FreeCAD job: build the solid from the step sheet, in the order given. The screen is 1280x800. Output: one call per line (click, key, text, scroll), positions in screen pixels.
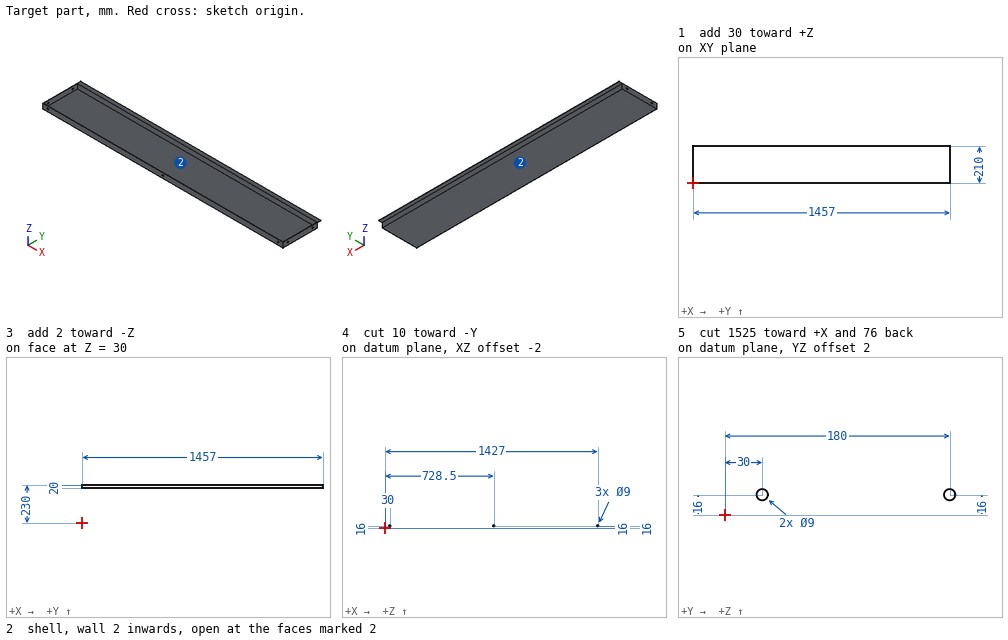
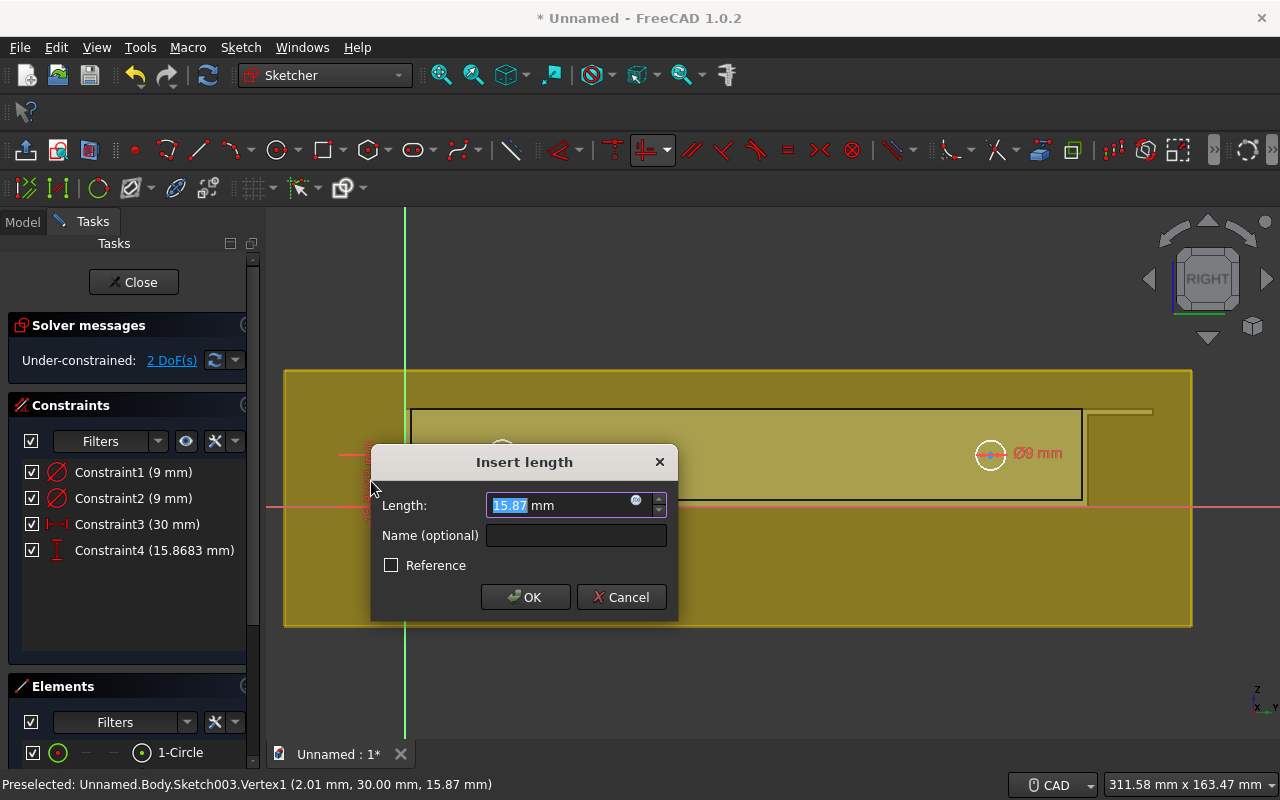
text(16)
key(Return)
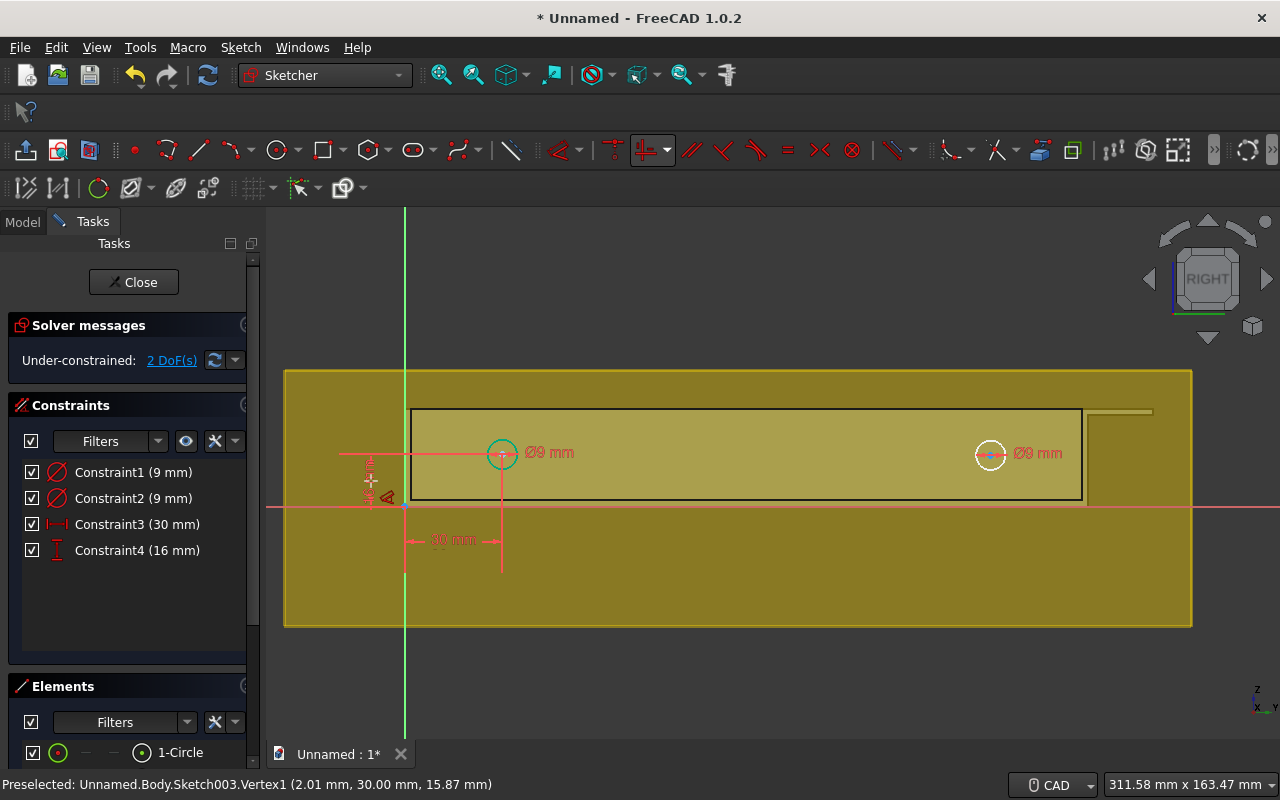
click(991, 455)
click(1025, 481)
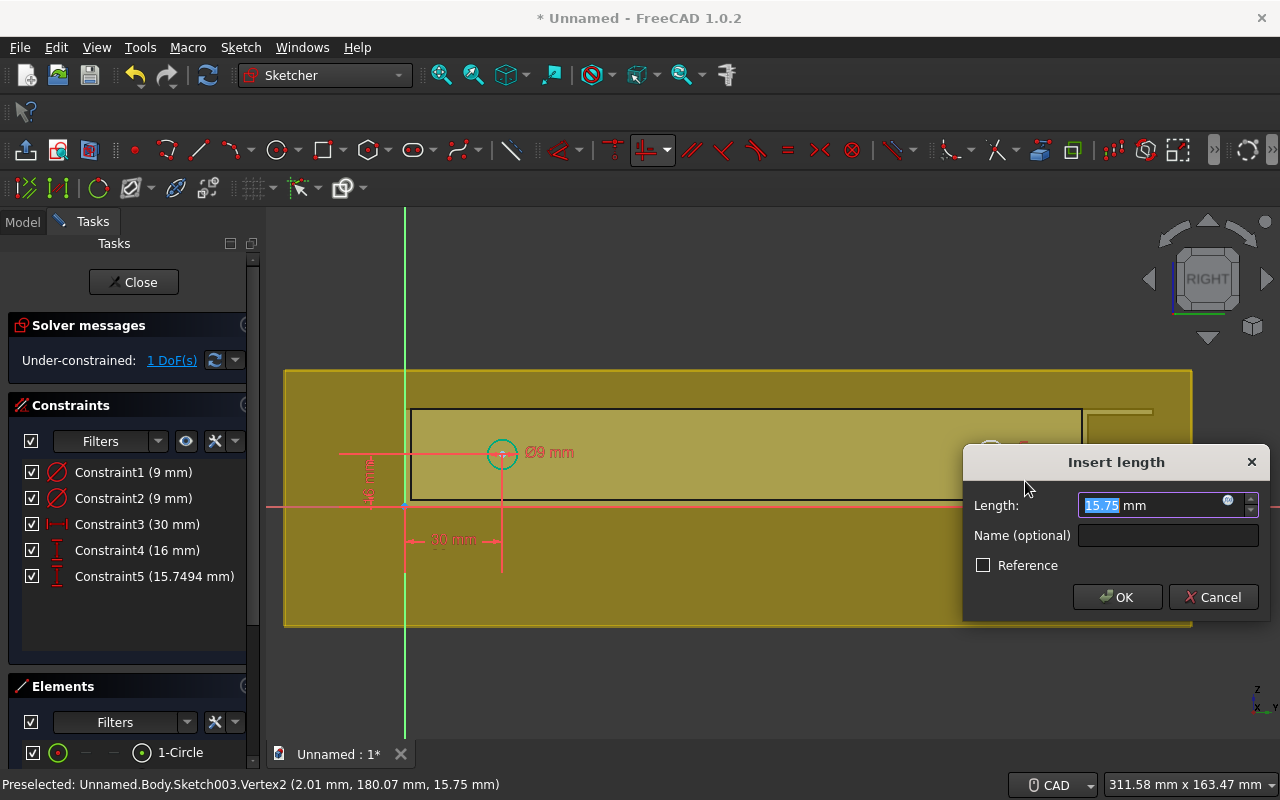
text(16)
key(Return)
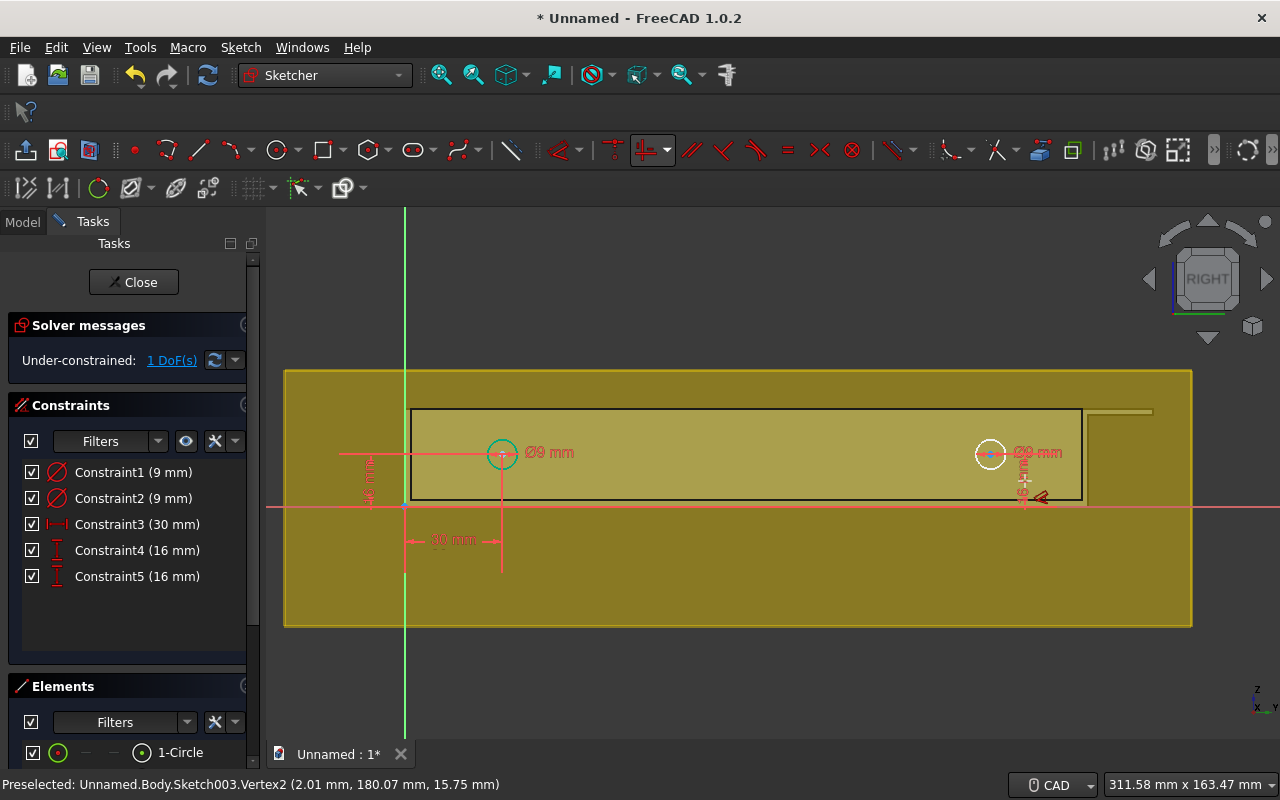
click(991, 454)
click(698, 541)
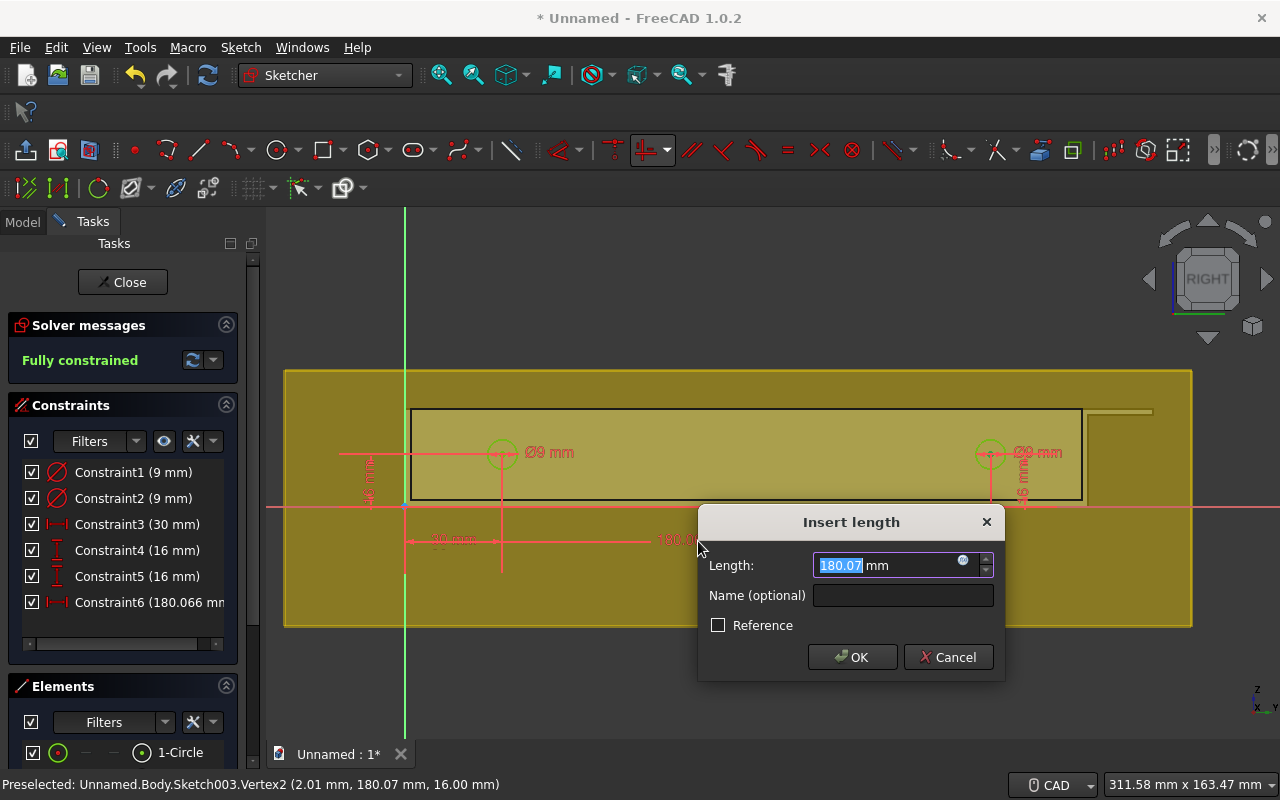
text(180)
key(Return)
key(Escape)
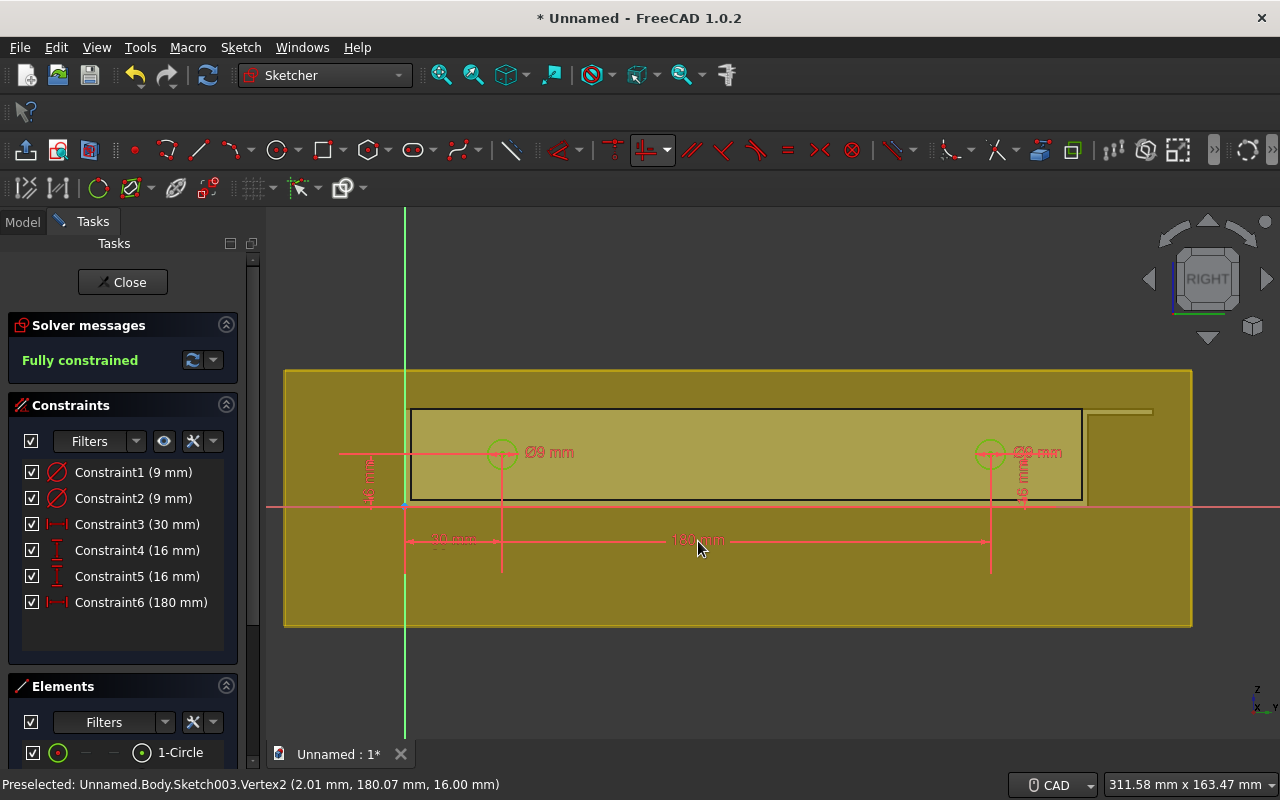
click(123, 282)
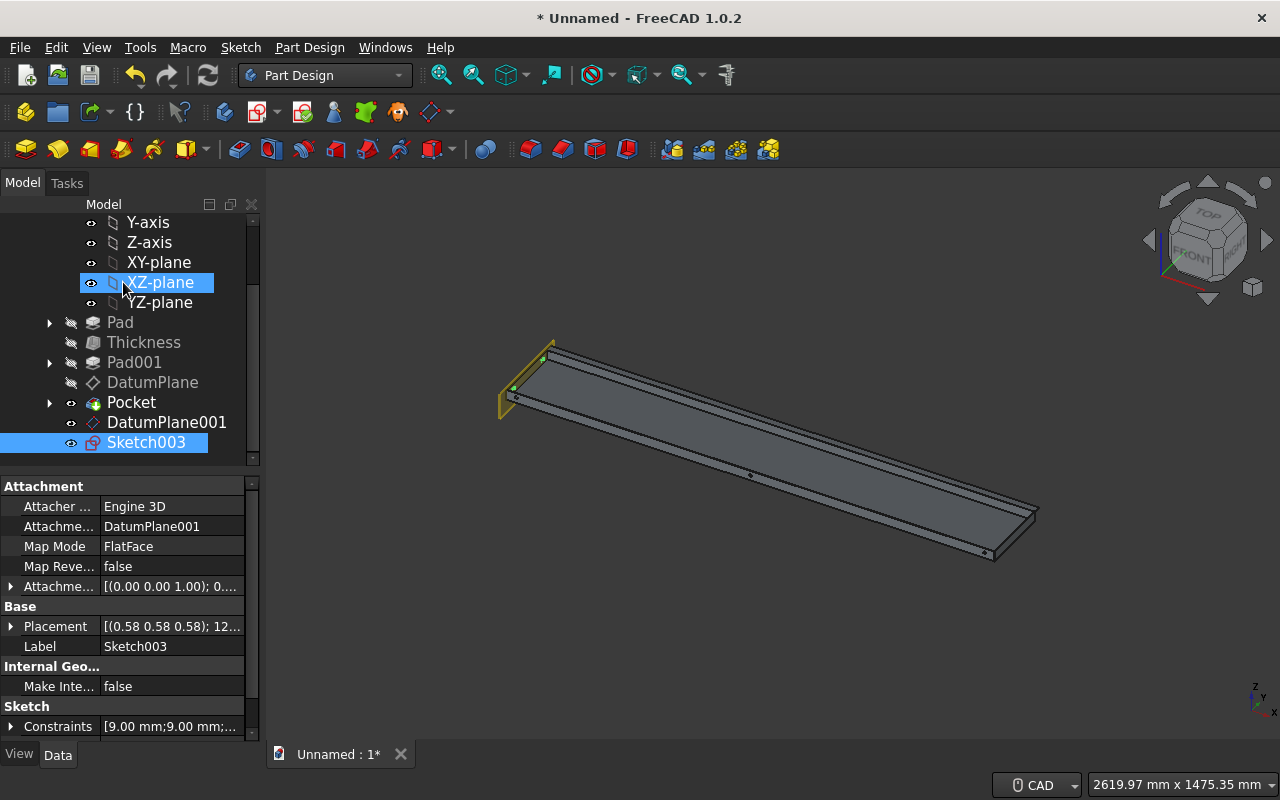
click(240, 150)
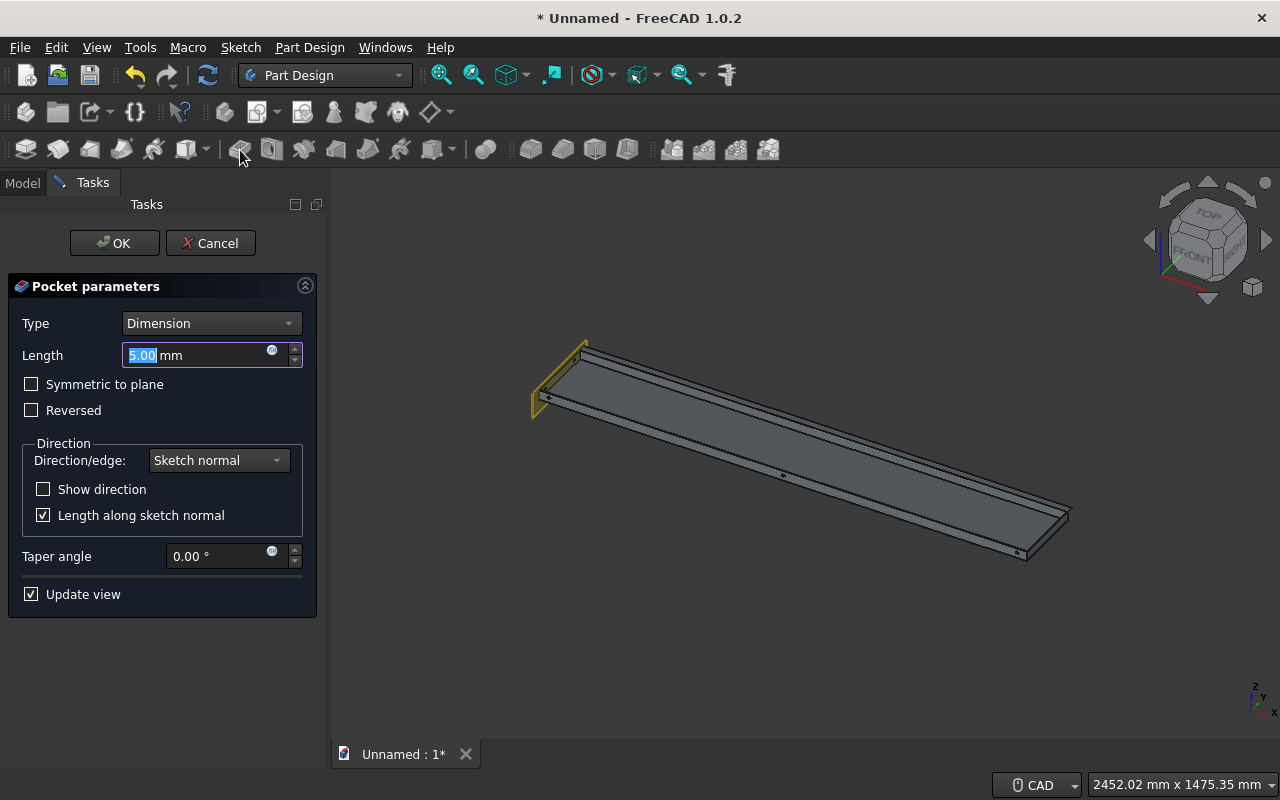
click(212, 324)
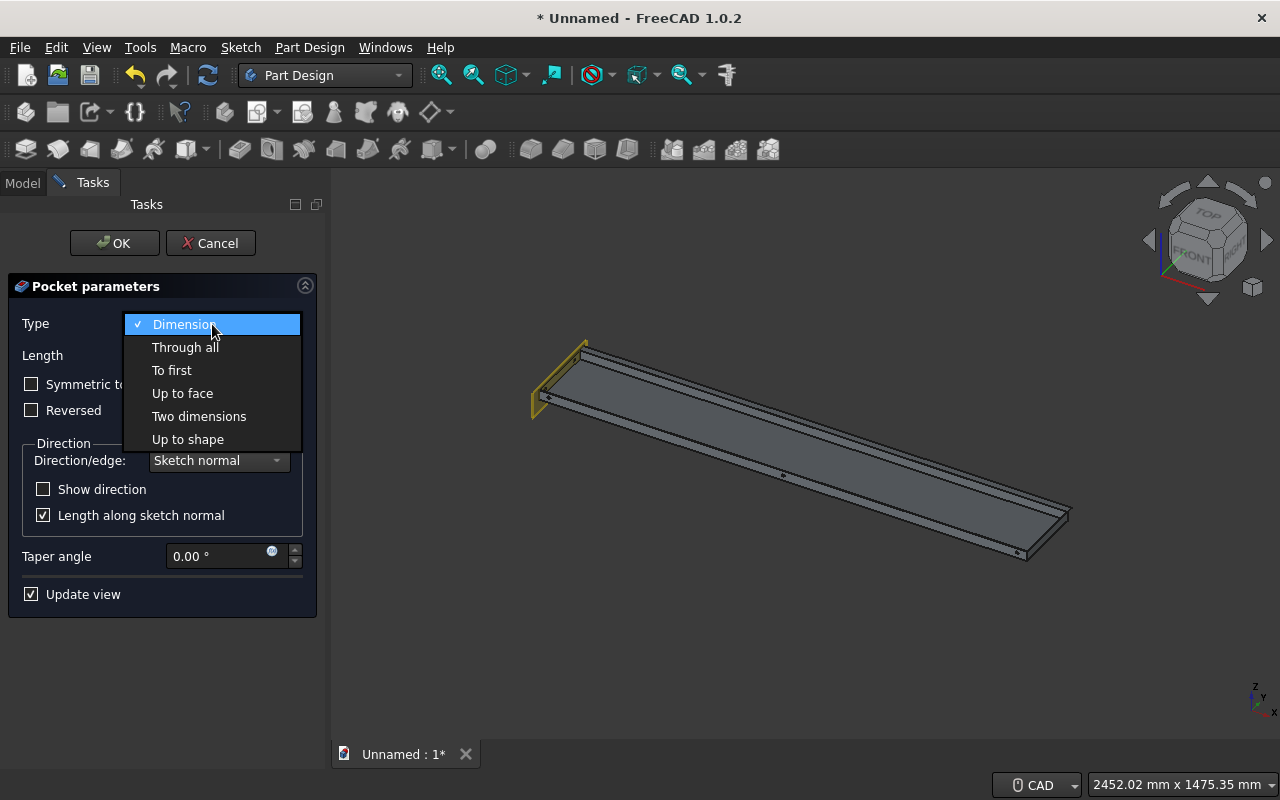
click(212, 416)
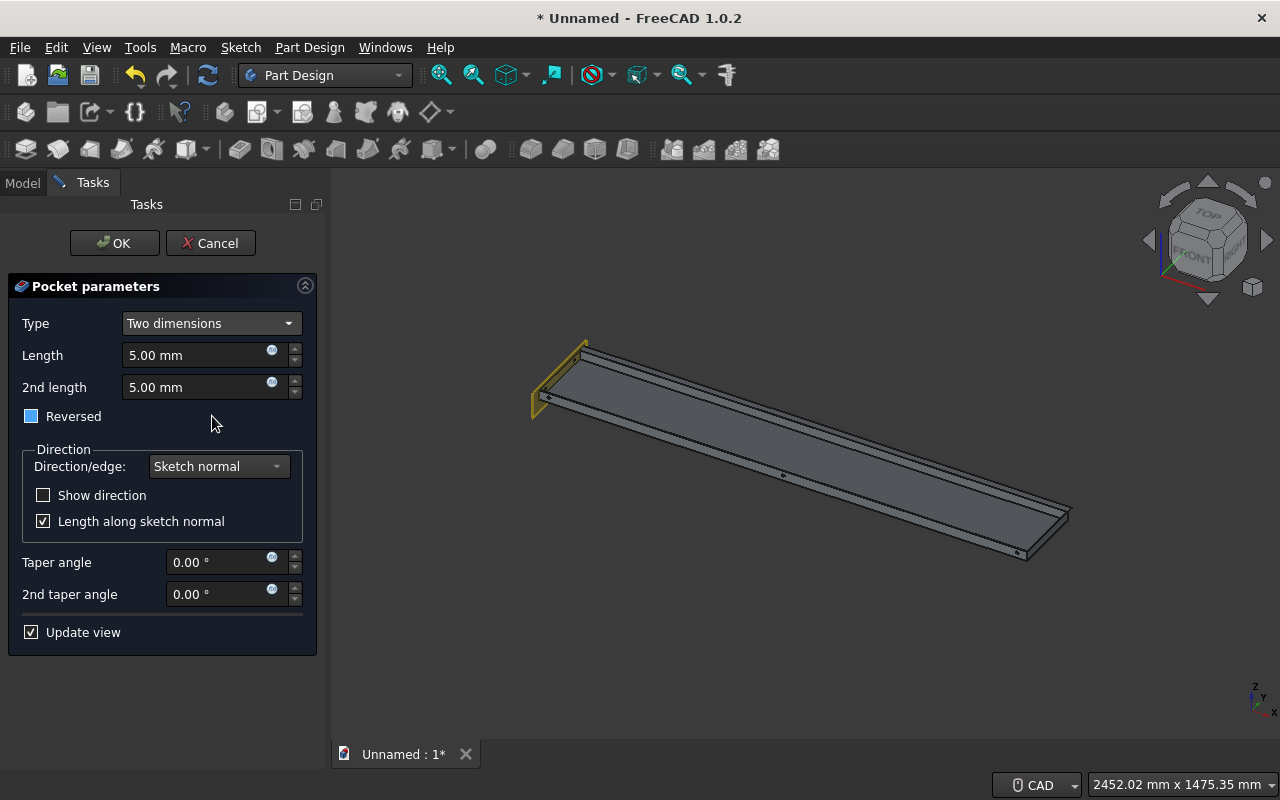
triple_click(204, 355)